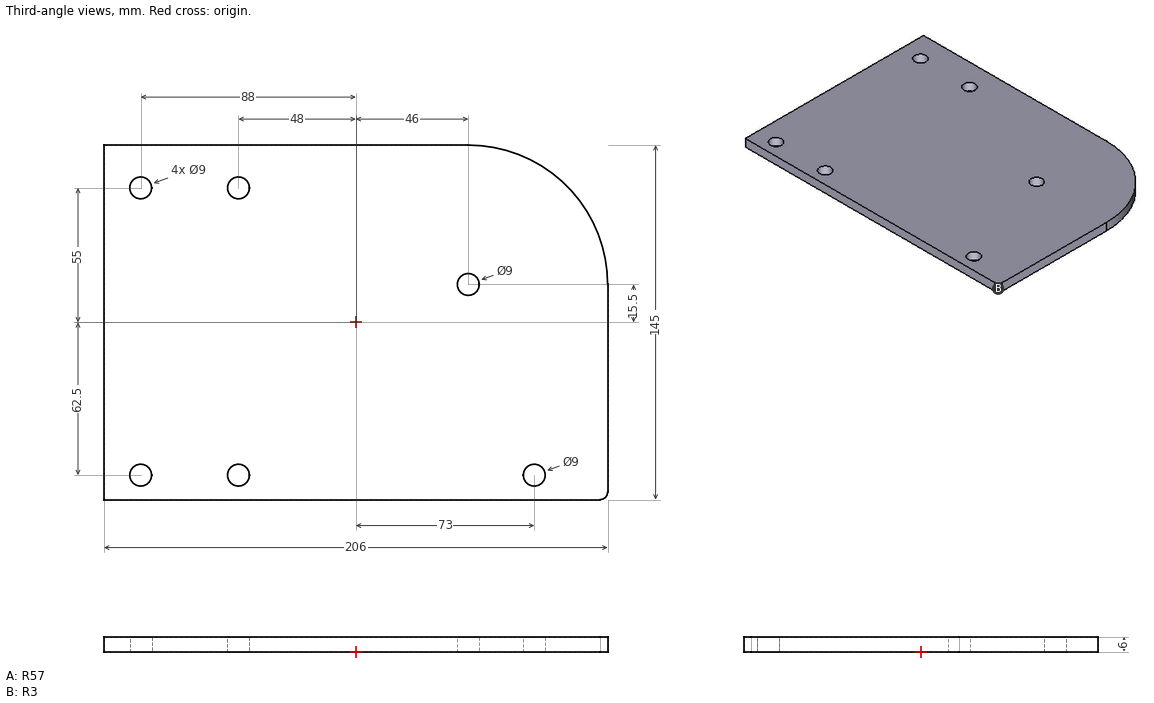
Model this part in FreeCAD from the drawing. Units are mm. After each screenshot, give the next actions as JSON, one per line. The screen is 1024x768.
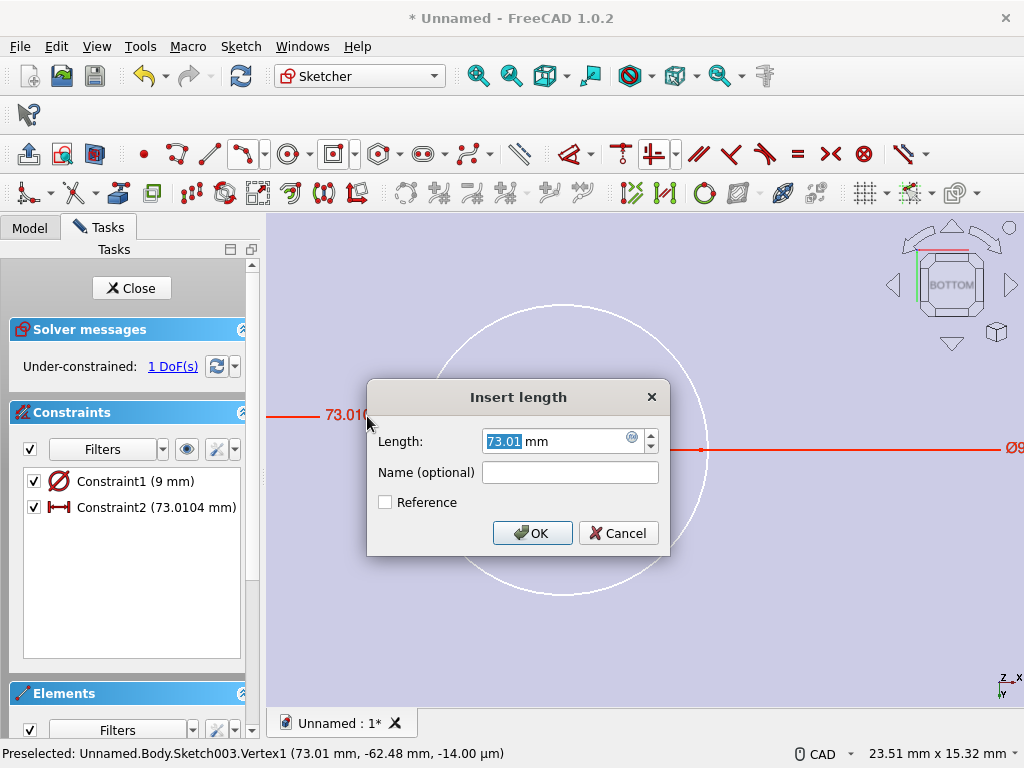
{"action": "type", "text": "73"}
{"action": "key", "text": "Return"}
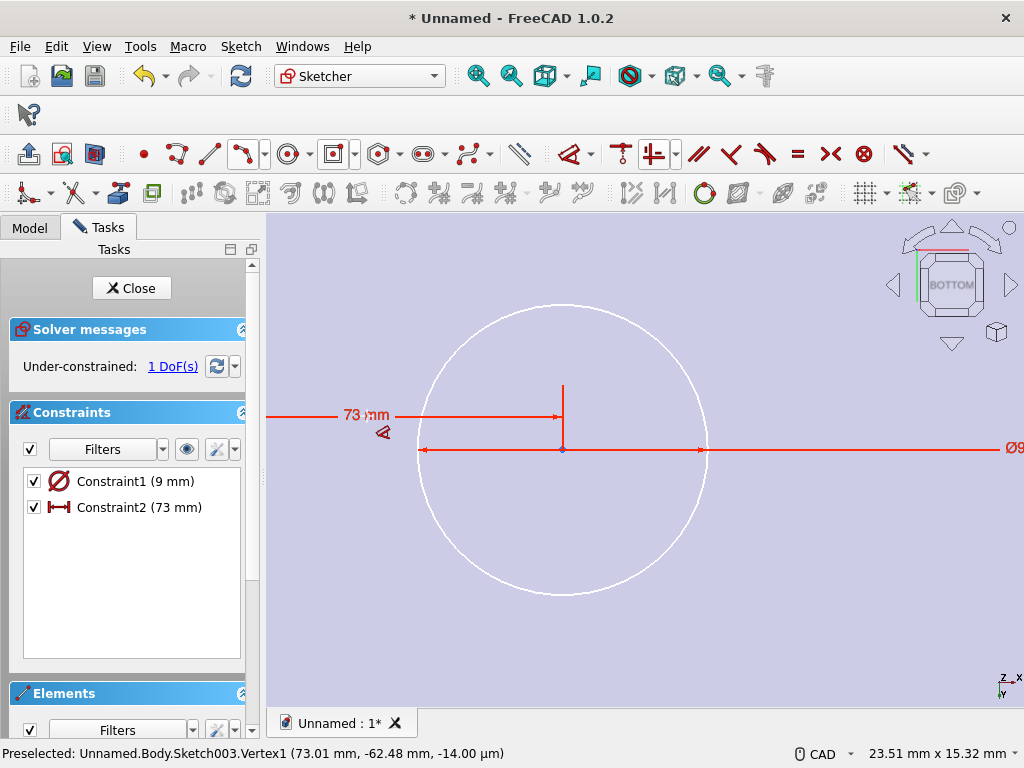
{"action": "left_click", "coordinate": [563, 450]}
{"action": "left_click", "coordinate": [597, 564]}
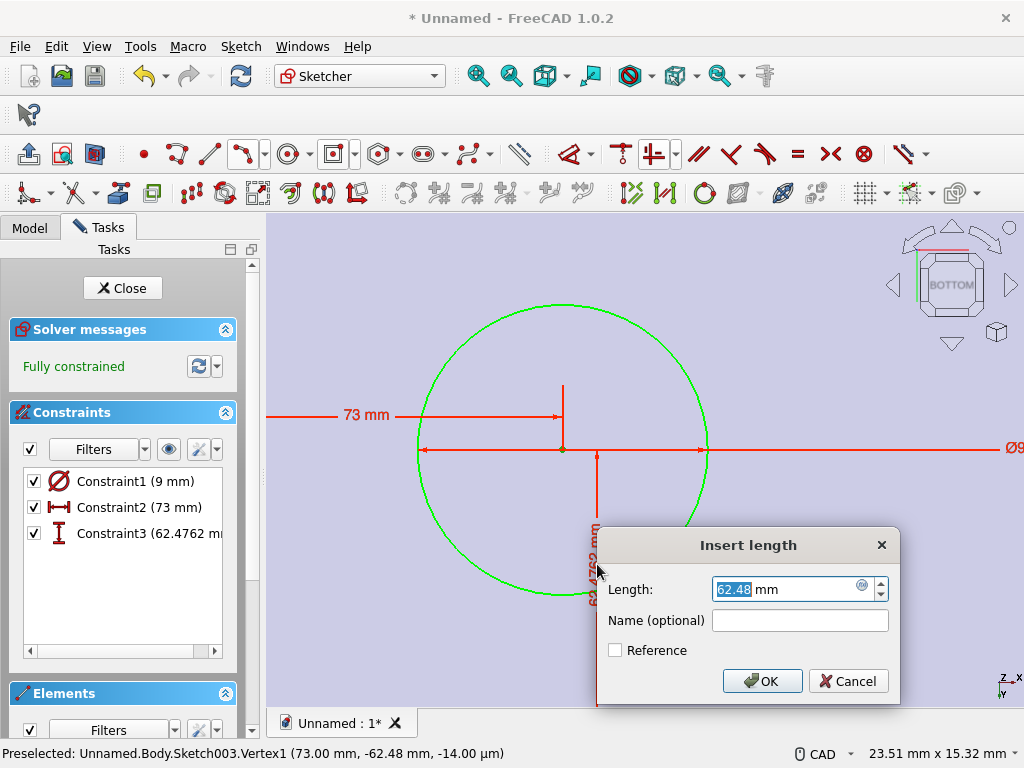
{"action": "type", "text": "62.5"}
{"action": "key", "text": "Return"}
{"action": "key", "text": "Escape"}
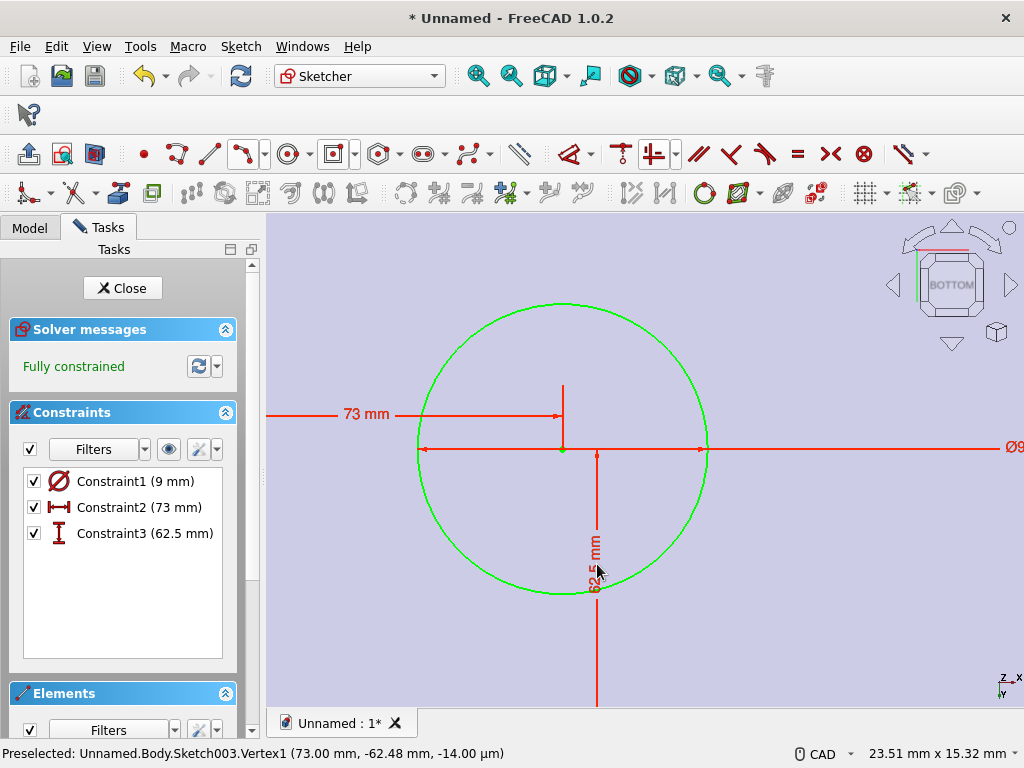
{"action": "left_click", "coordinate": [123, 288]}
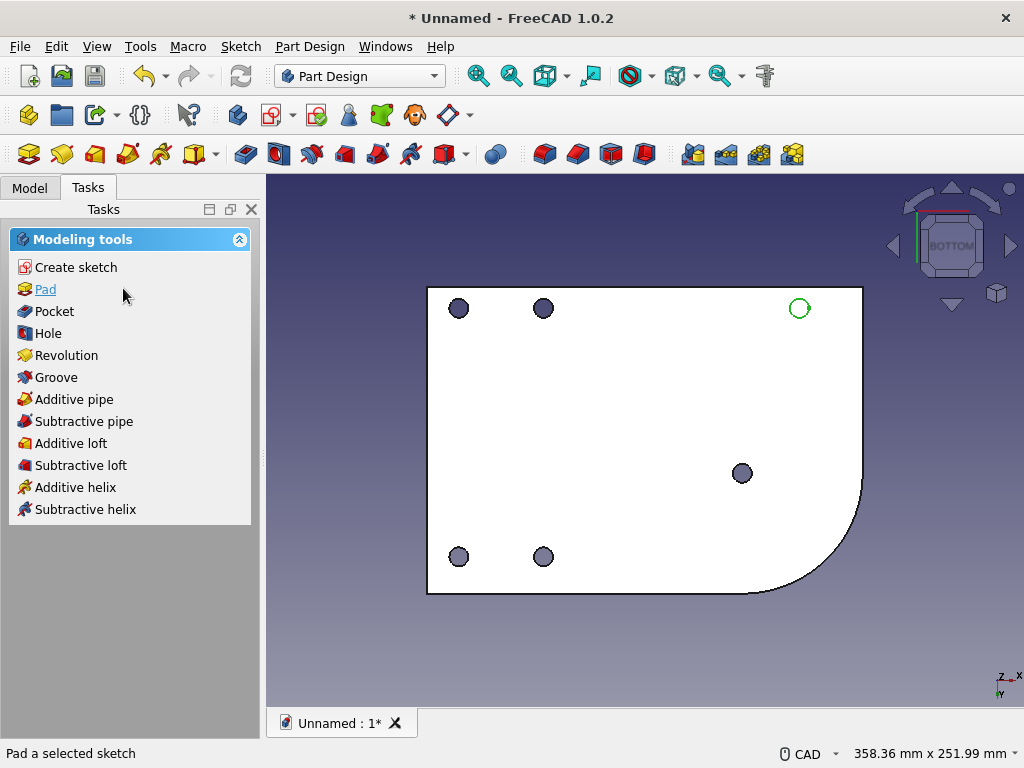
{"action": "left_click", "coordinate": [246, 154]}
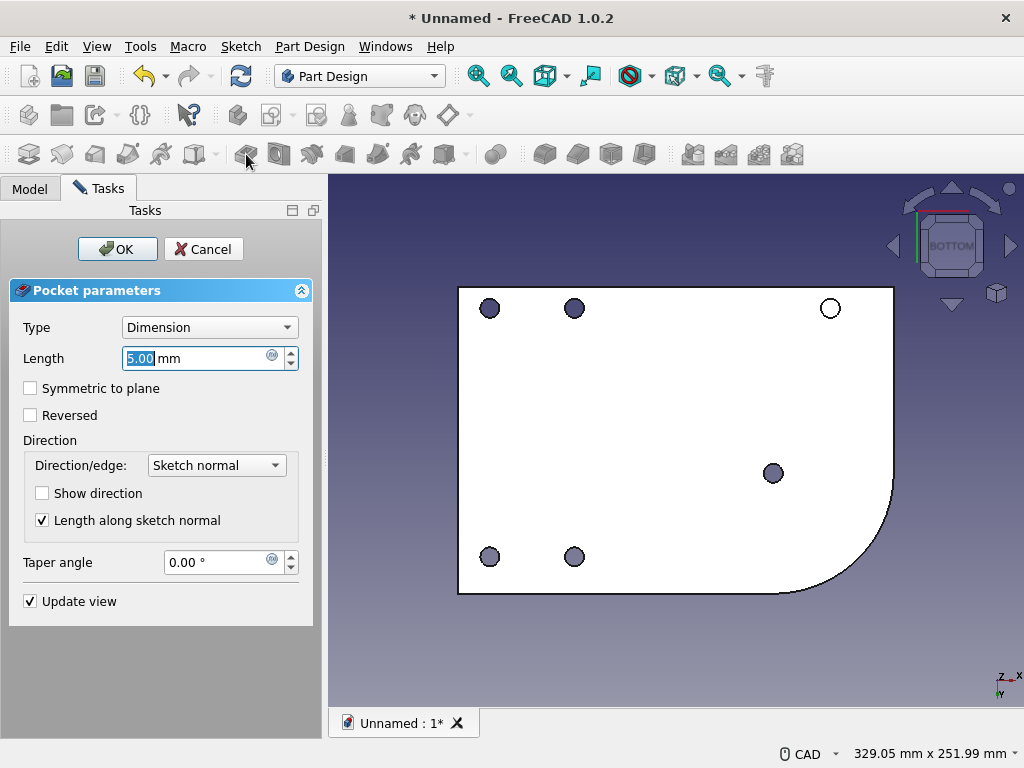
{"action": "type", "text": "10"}
{"action": "key", "text": "Tab"}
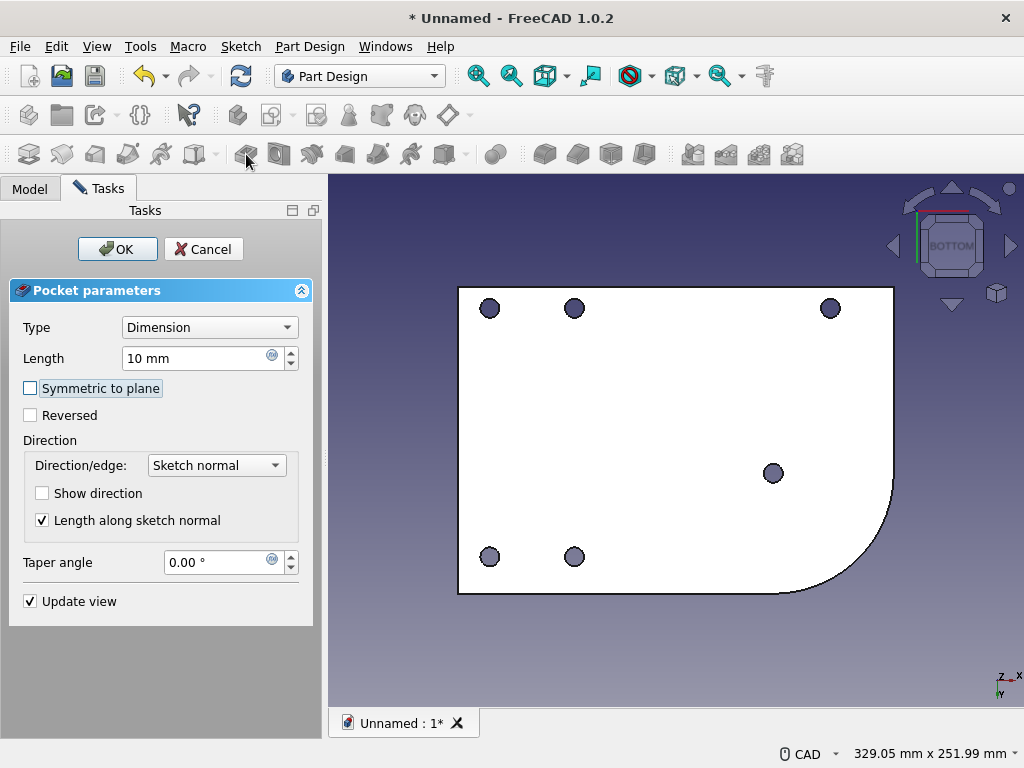
{"action": "left_click", "coordinate": [118, 249]}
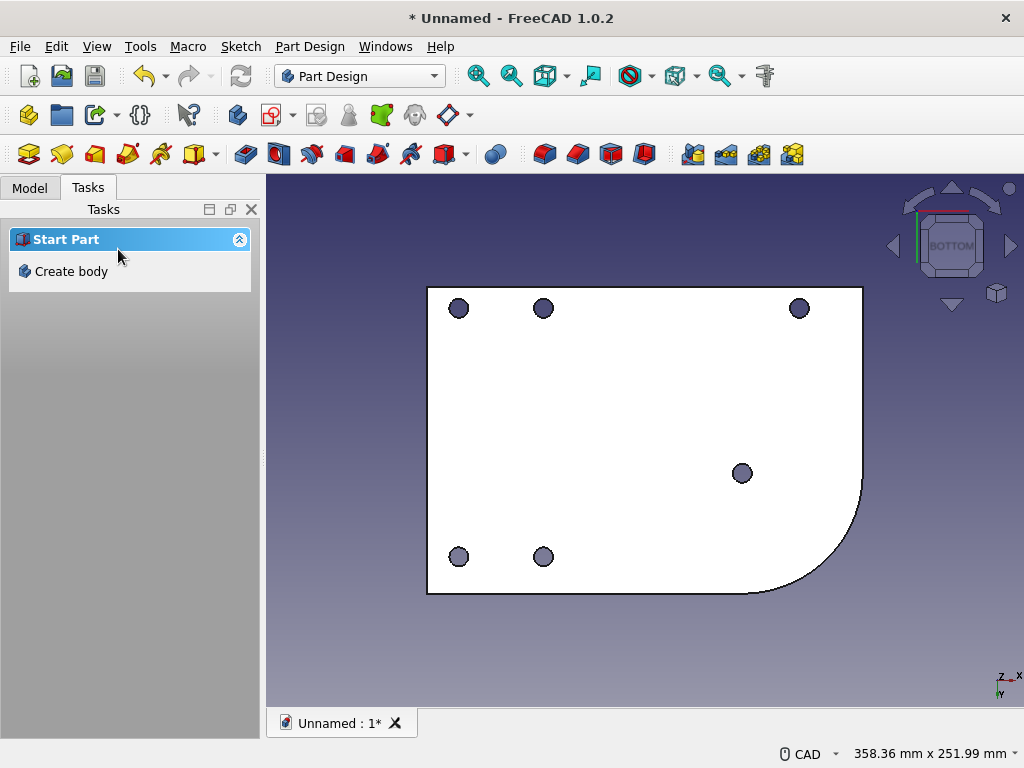
{"action": "key", "text": "0"}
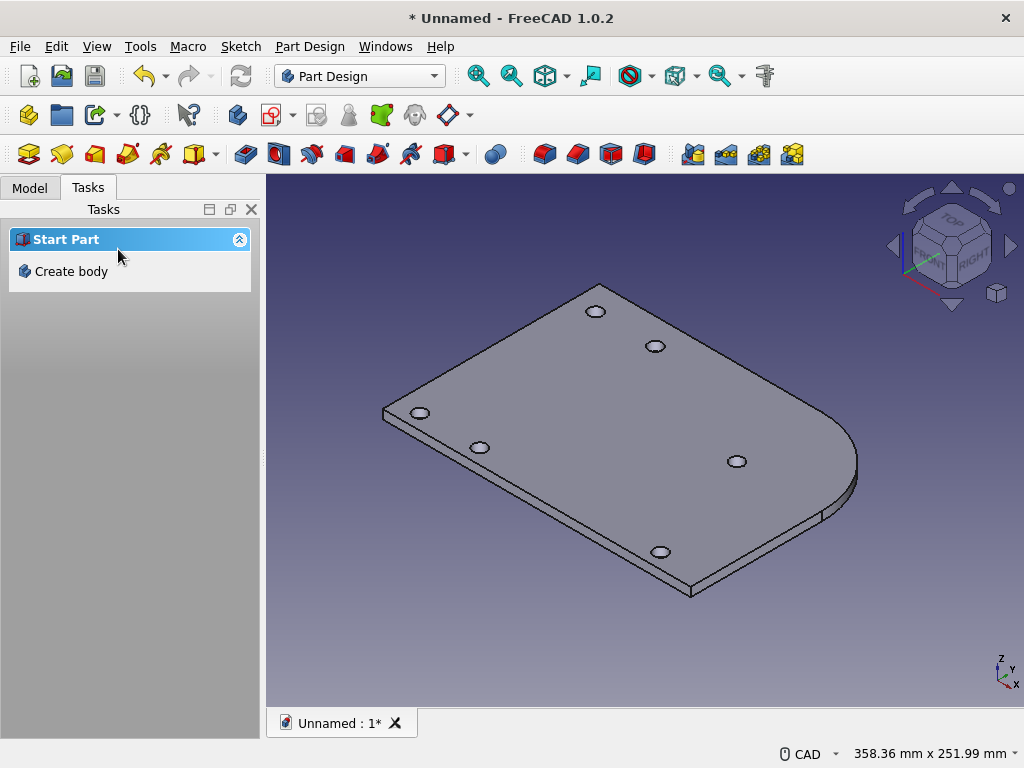
{"action": "left_click", "coordinate": [691, 592]}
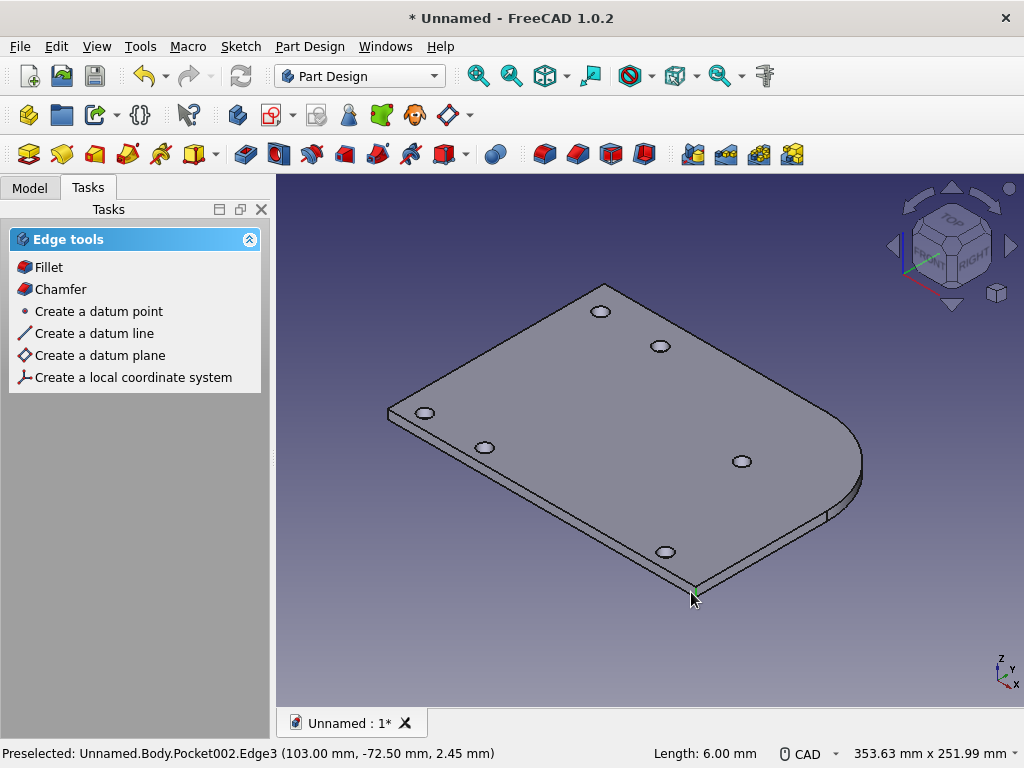
{"action": "left_click", "coordinate": [545, 154]}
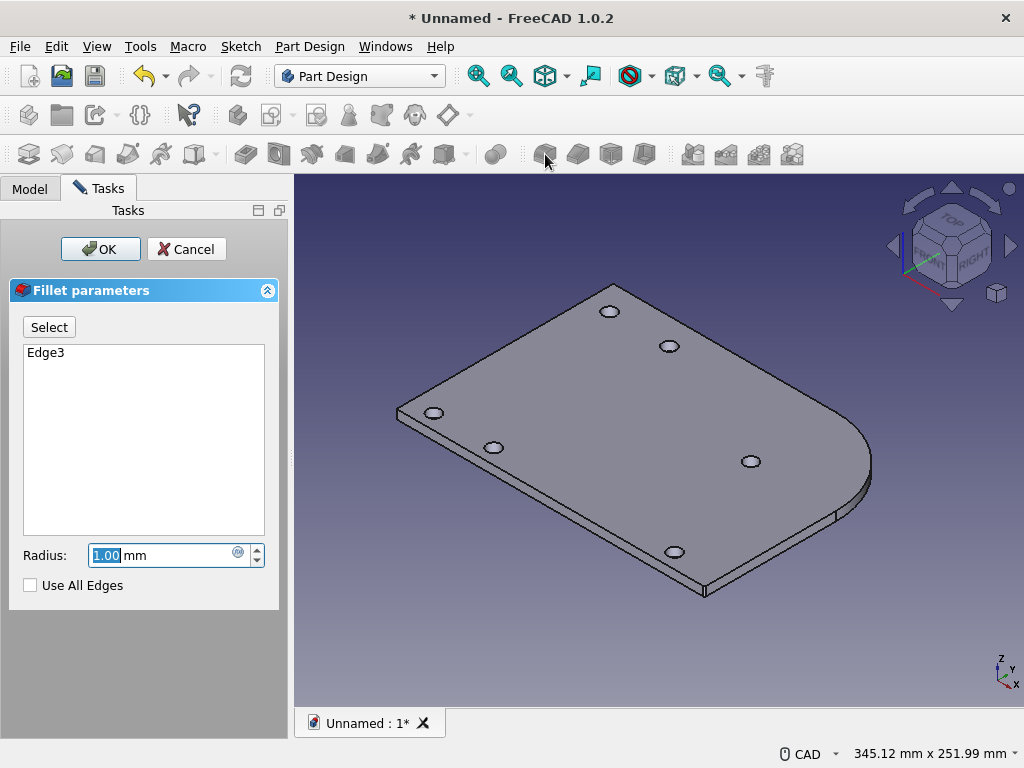
{"action": "type", "text": "3"}
{"action": "key", "text": "Tab"}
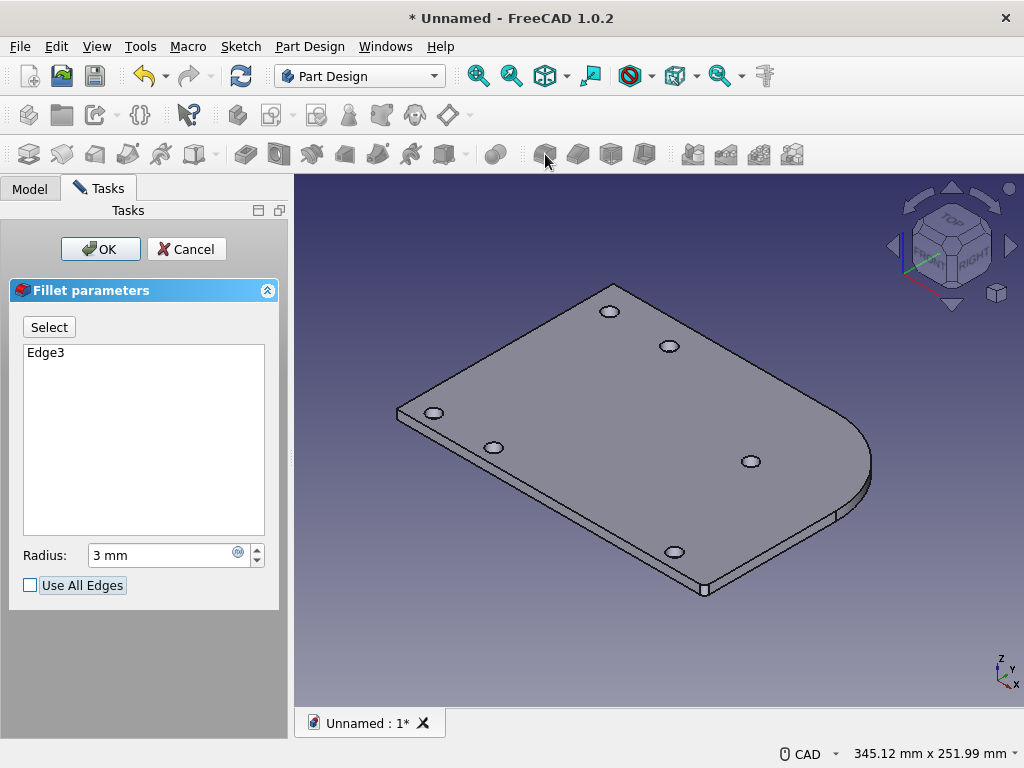
{"action": "left_click", "coordinate": [101, 249]}